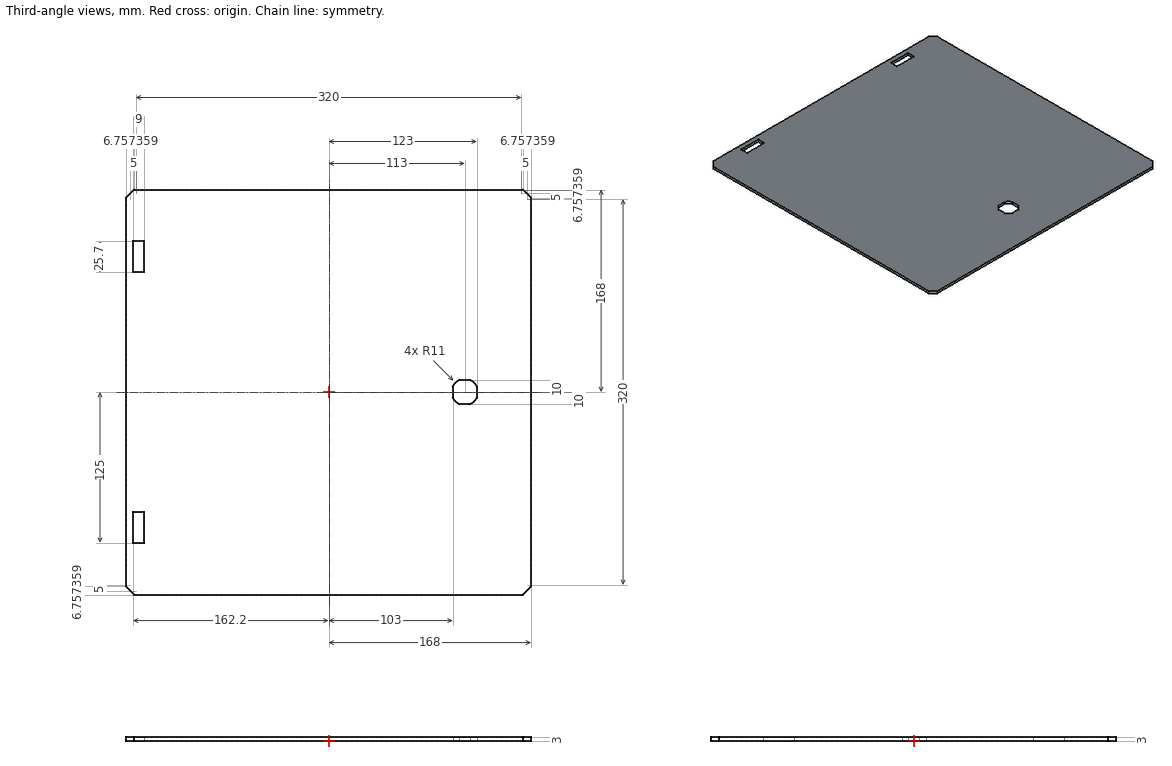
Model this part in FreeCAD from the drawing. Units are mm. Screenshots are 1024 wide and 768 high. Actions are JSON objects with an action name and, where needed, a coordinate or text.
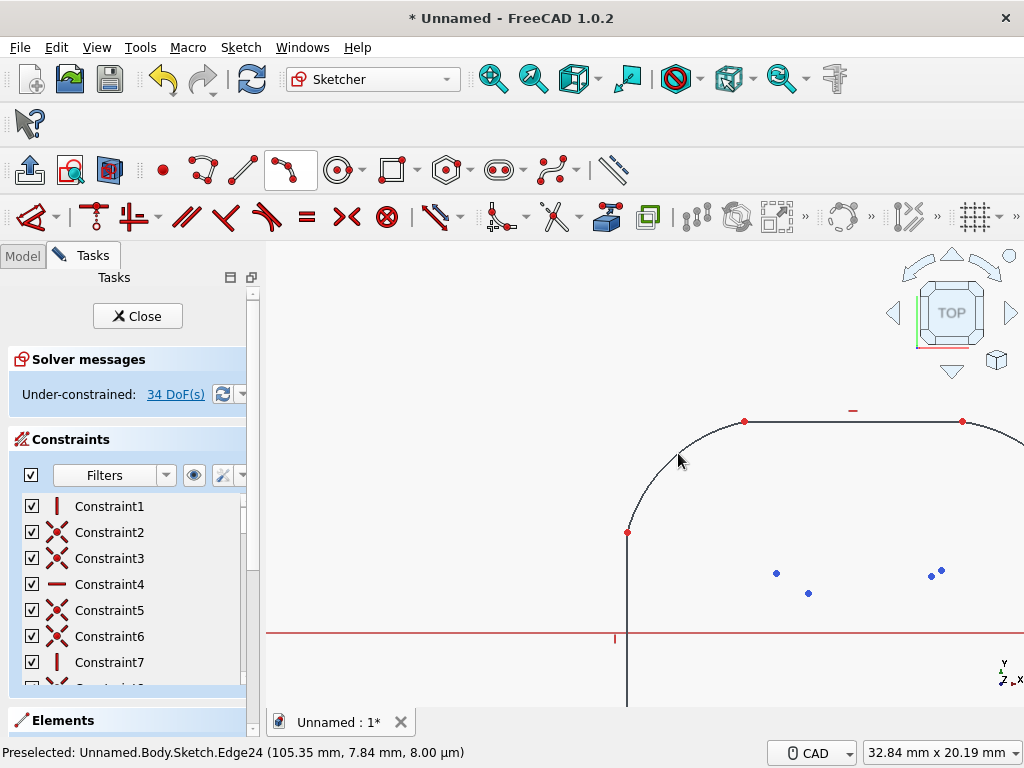
{"action": "scroll", "coordinate": [675, 467], "scroll_direction": "down", "scroll_amount": 16}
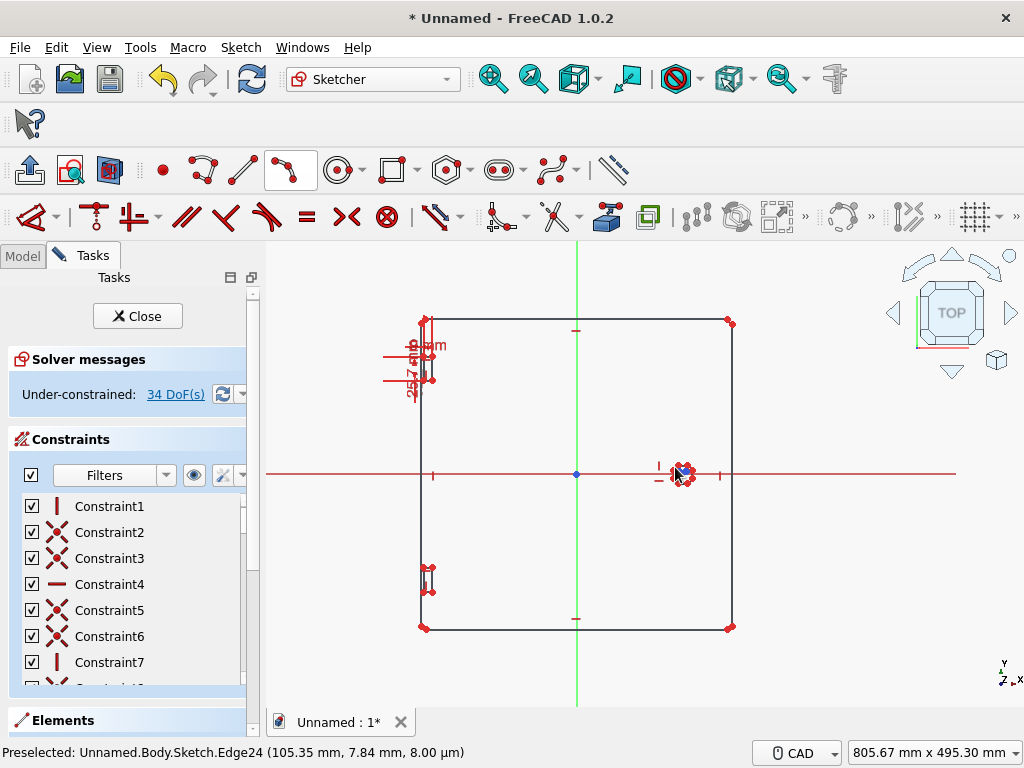
{"action": "scroll", "coordinate": [691, 468], "scroll_direction": "up", "scroll_amount": 10}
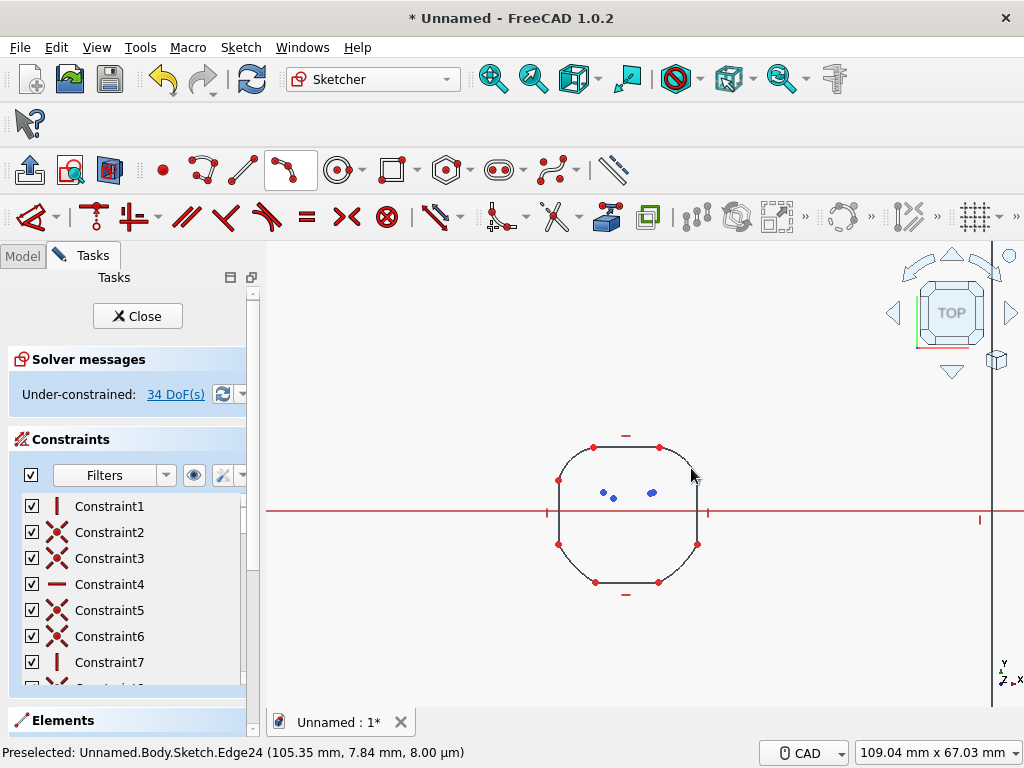
{"action": "left_click", "coordinate": [690, 466]}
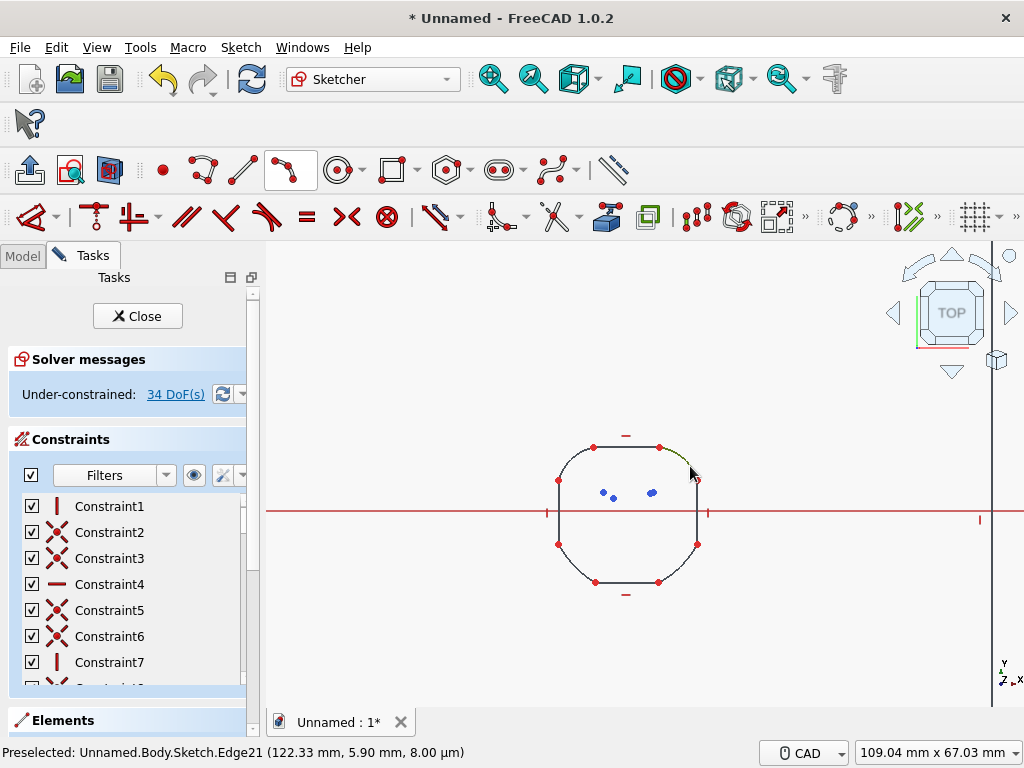
{"action": "left_click", "coordinate": [673, 574]}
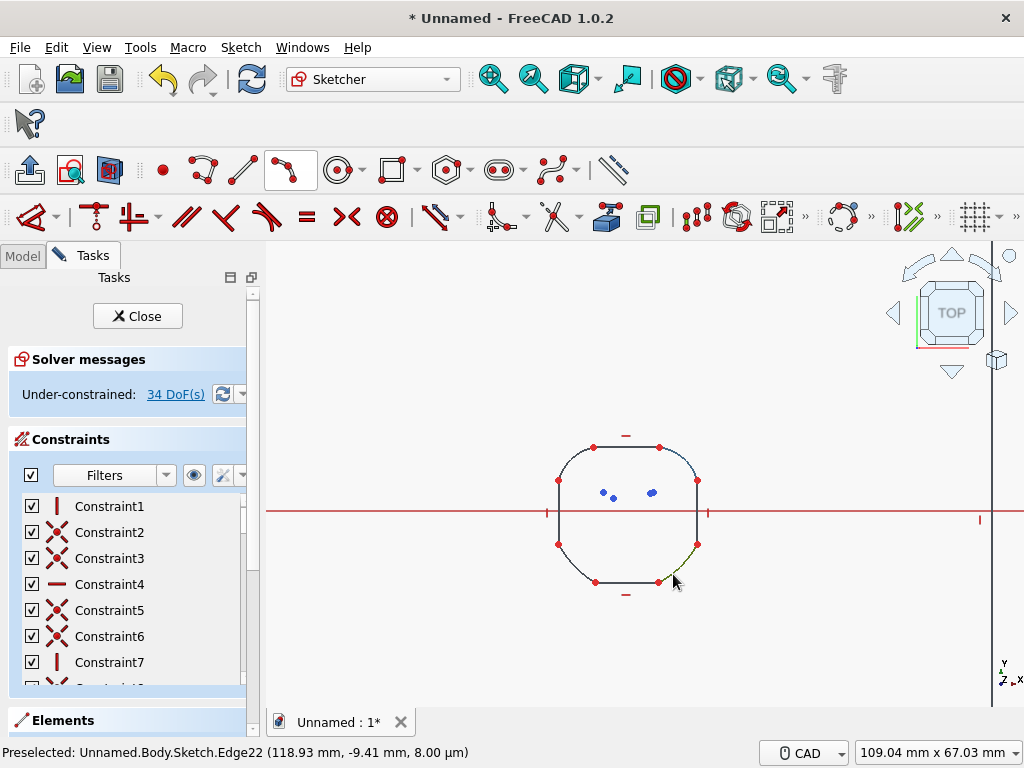
{"action": "left_click", "coordinate": [94, 218]}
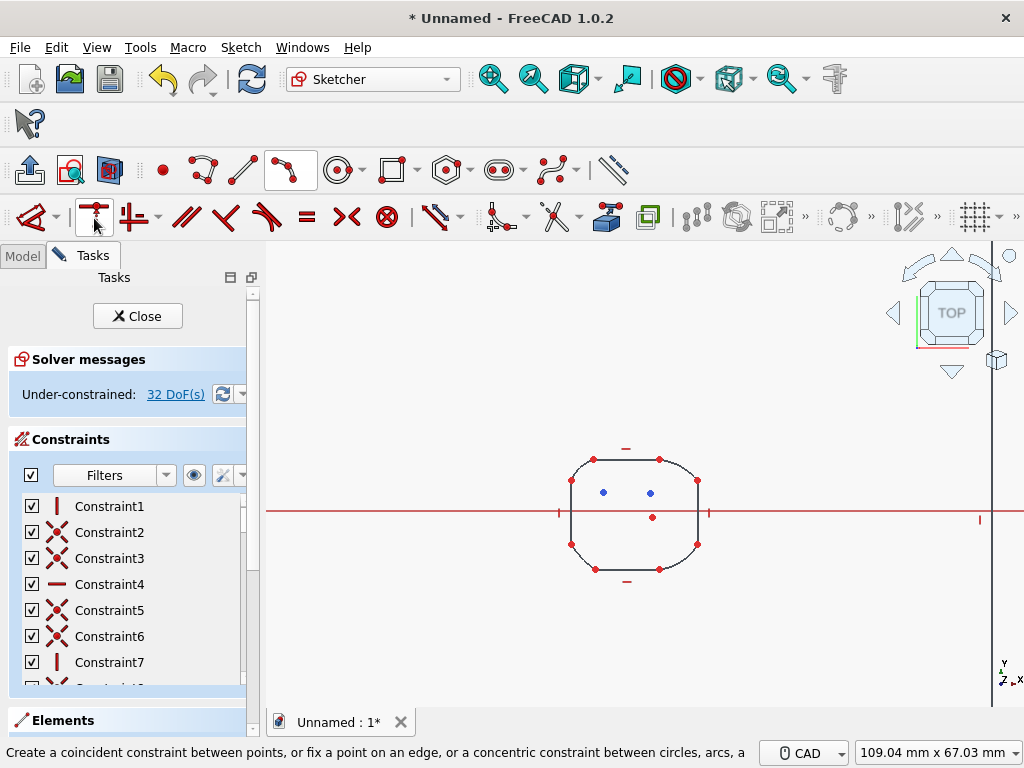
{"action": "left_click", "coordinate": [688, 471]}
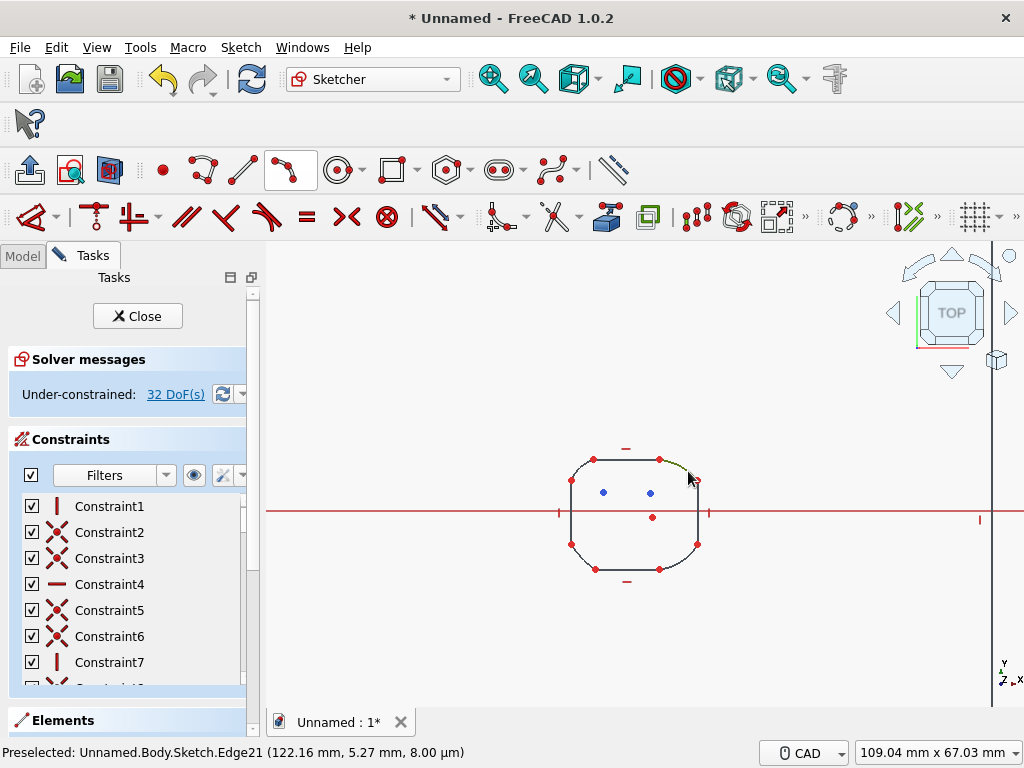
{"action": "scroll", "coordinate": [577, 553], "scroll_direction": "up", "scroll_amount": 2}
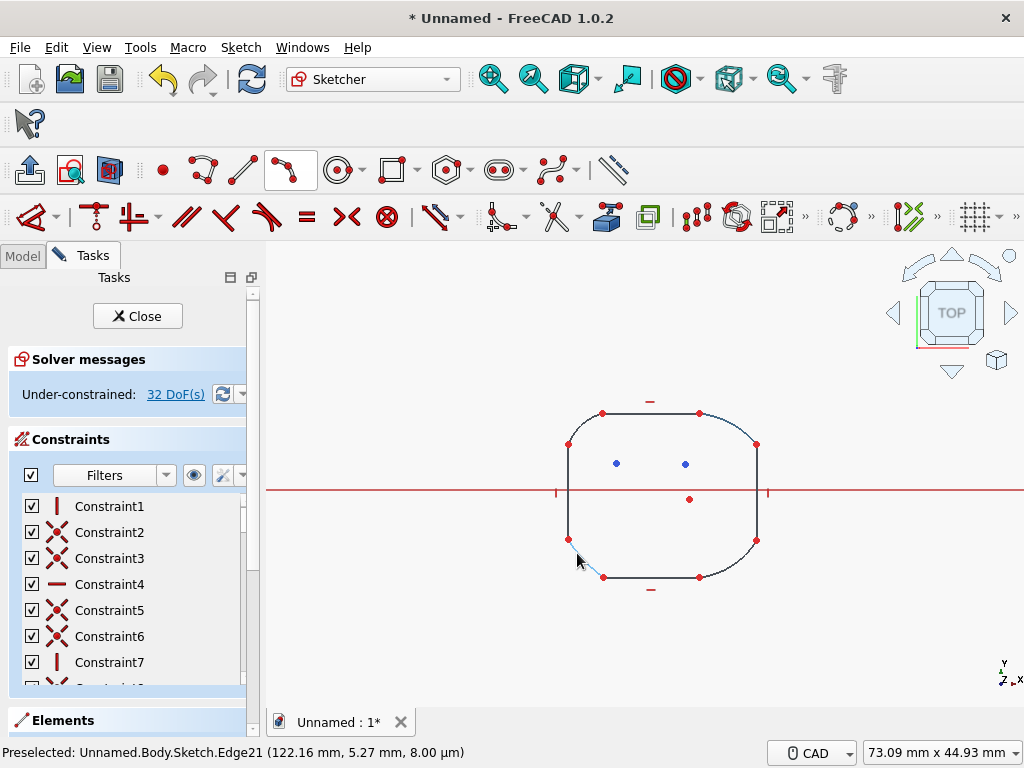
{"action": "left_click", "coordinate": [577, 553]}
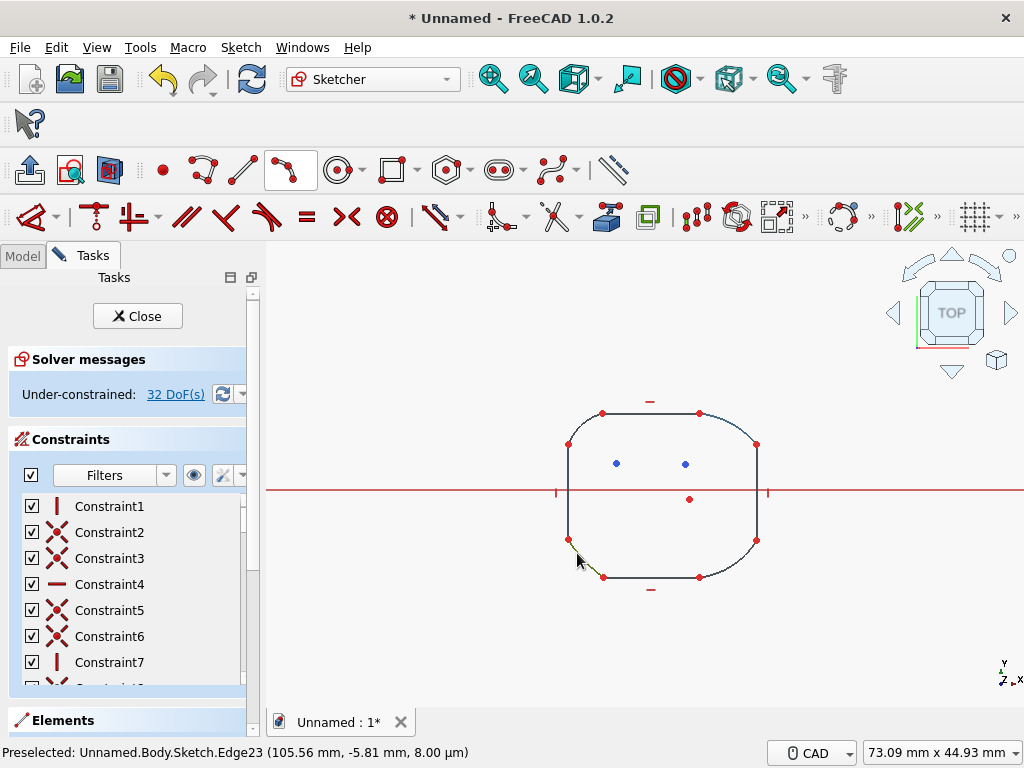
{"action": "left_click", "coordinate": [94, 218]}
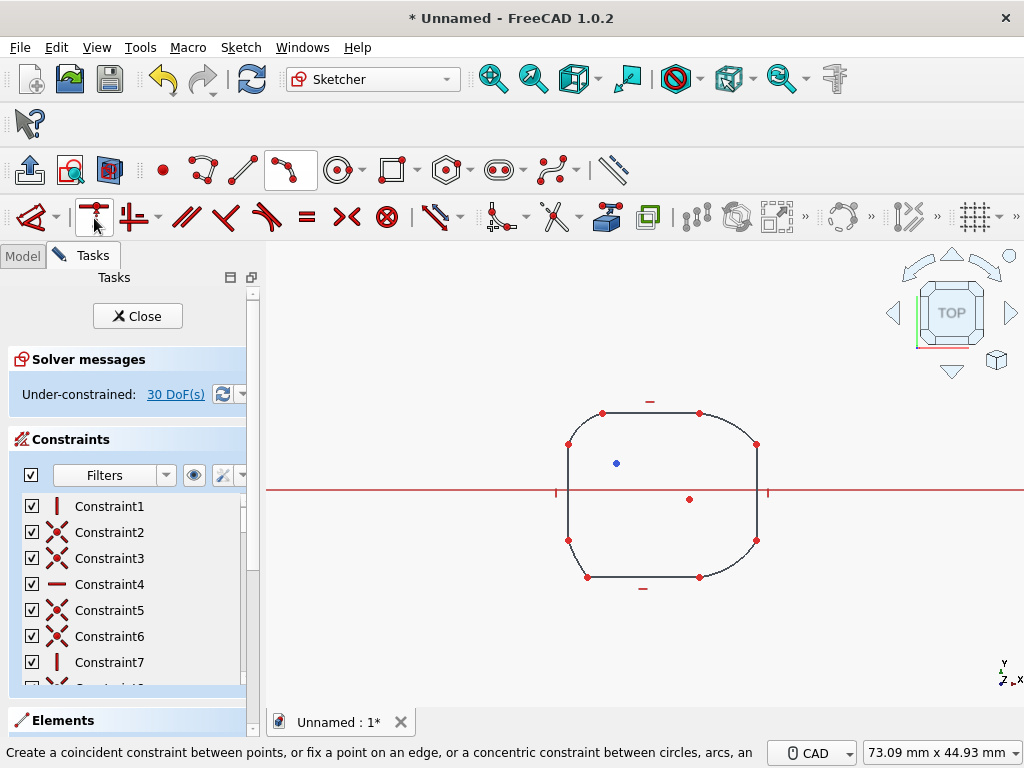
{"action": "left_click", "coordinate": [743, 431]}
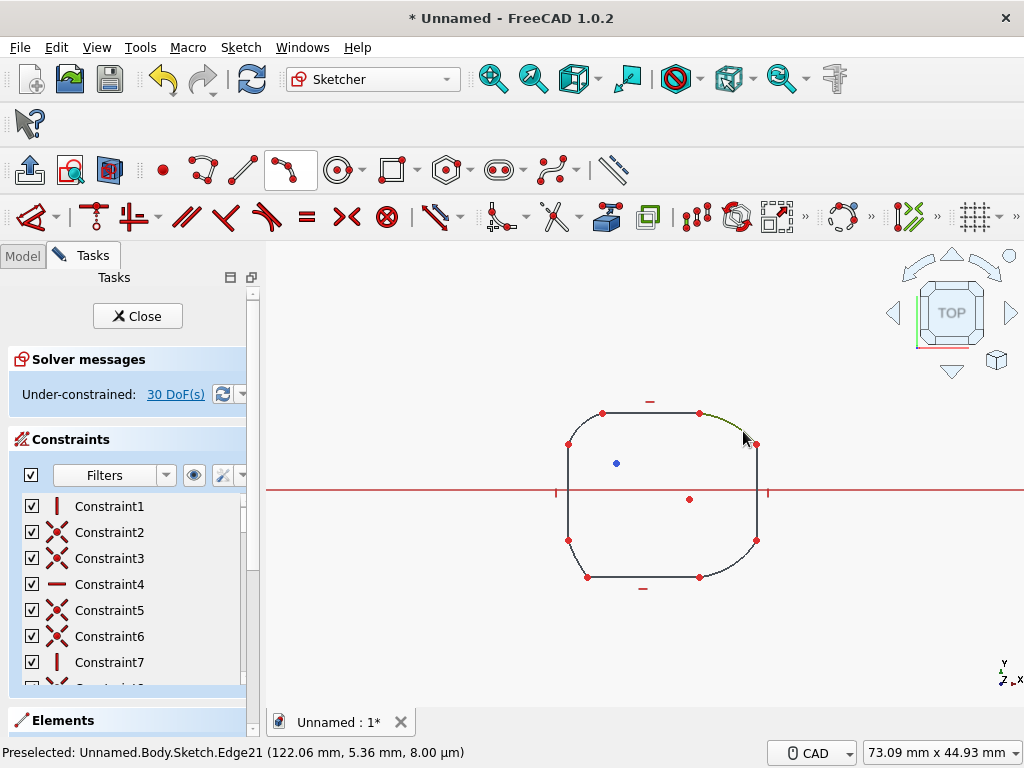
{"action": "left_click", "coordinate": [589, 419]}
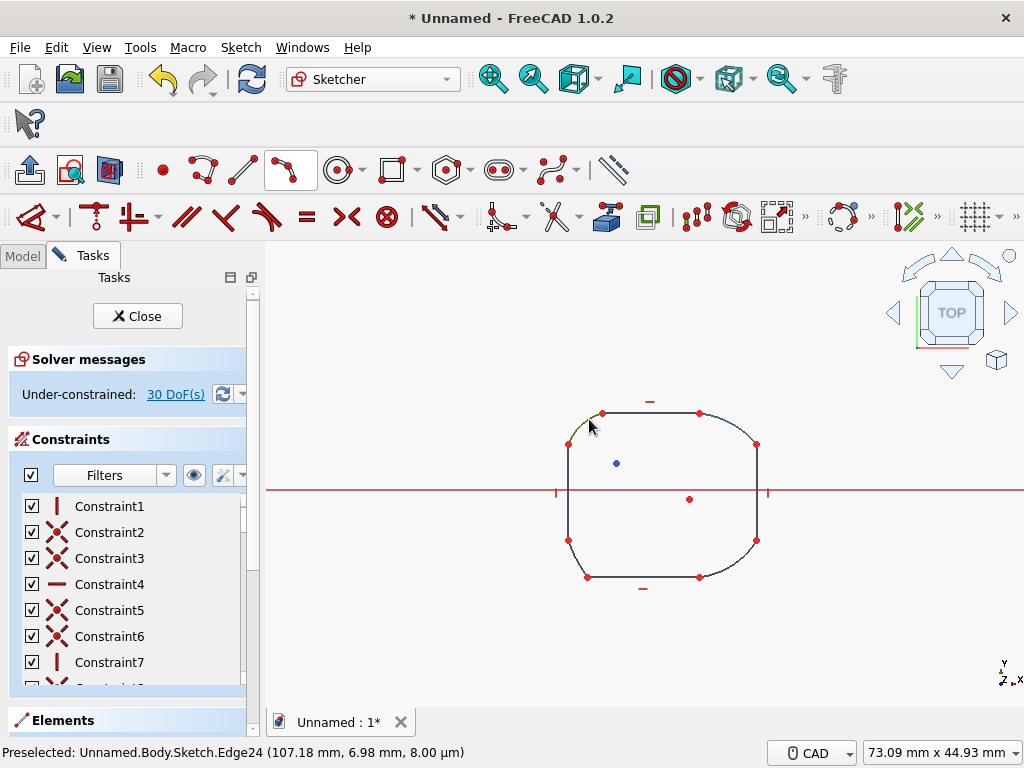
{"action": "left_click", "coordinate": [94, 218]}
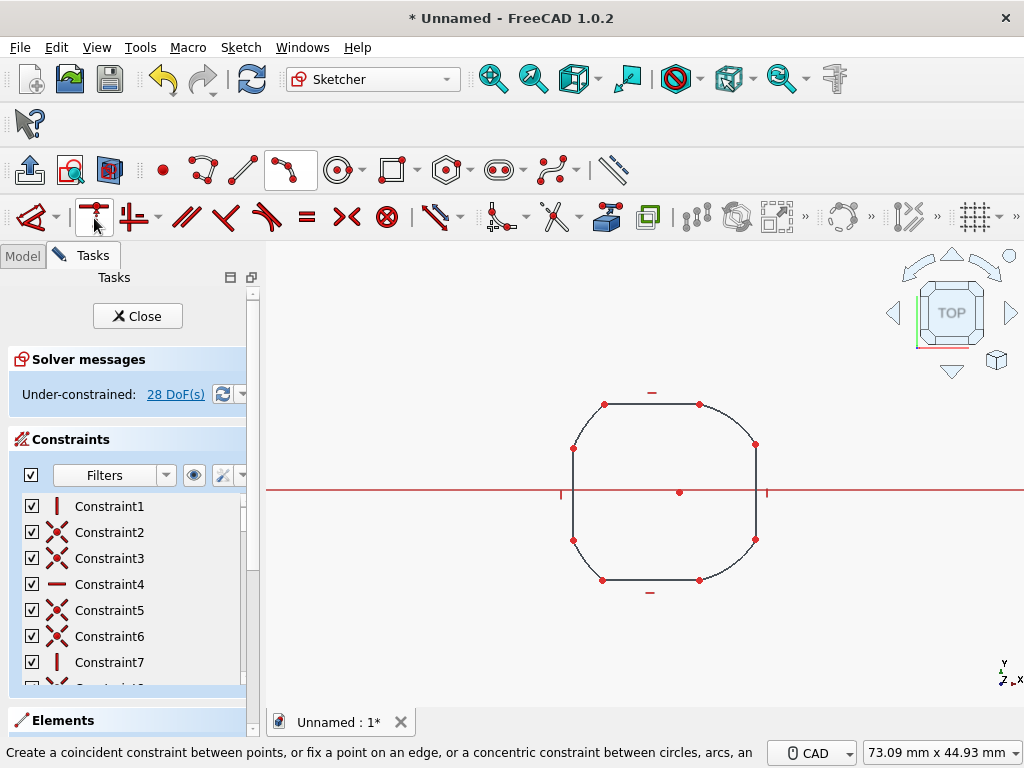
{"action": "left_click", "coordinate": [743, 428]}